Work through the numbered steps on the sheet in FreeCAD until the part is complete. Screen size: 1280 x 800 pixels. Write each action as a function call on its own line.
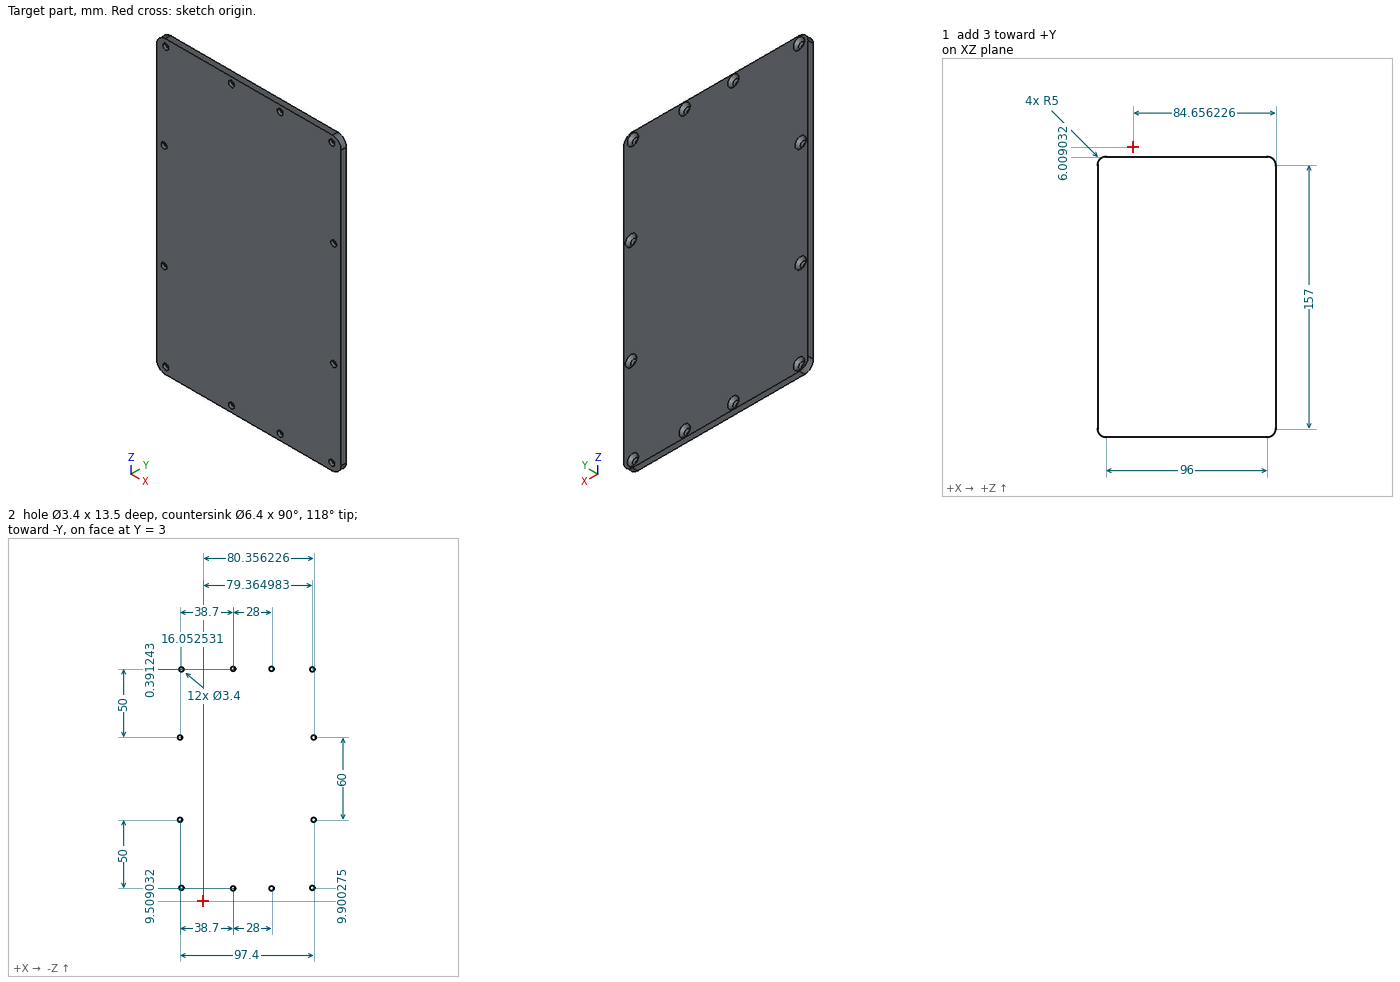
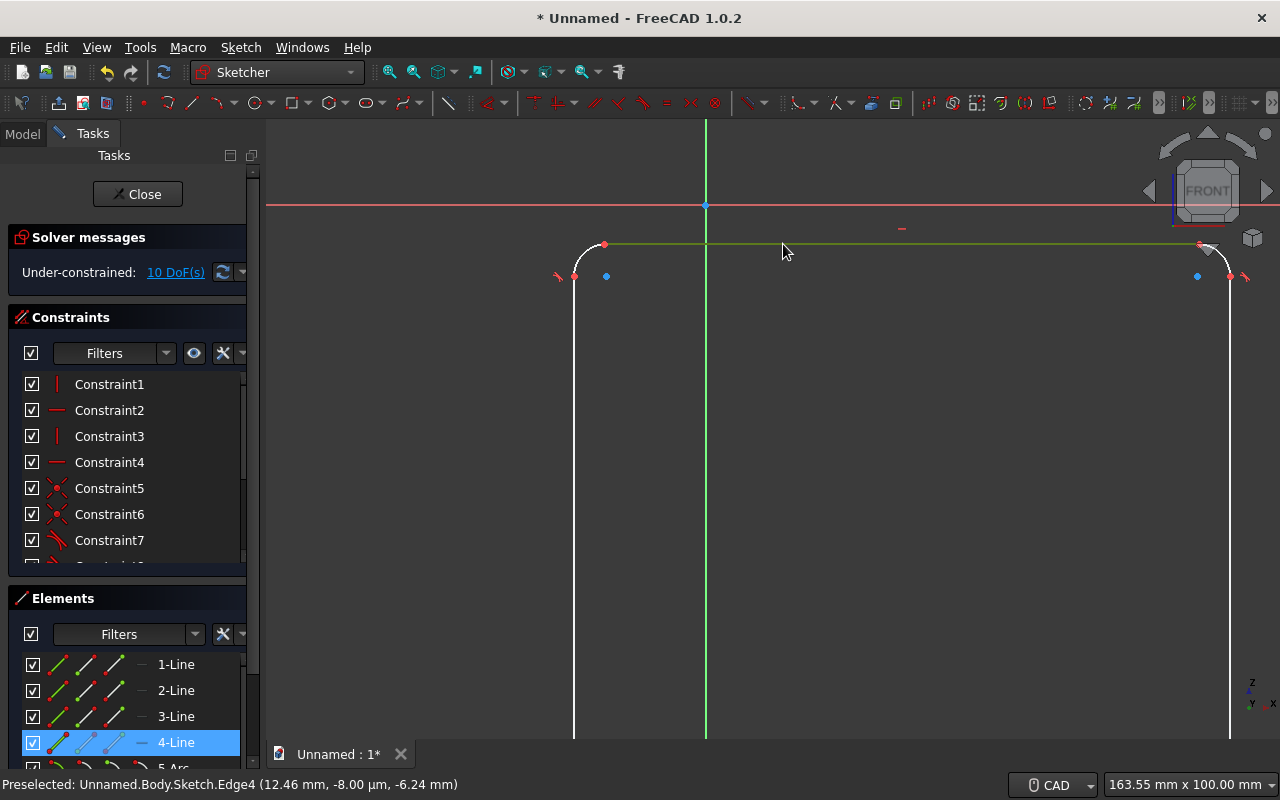
click(591, 248)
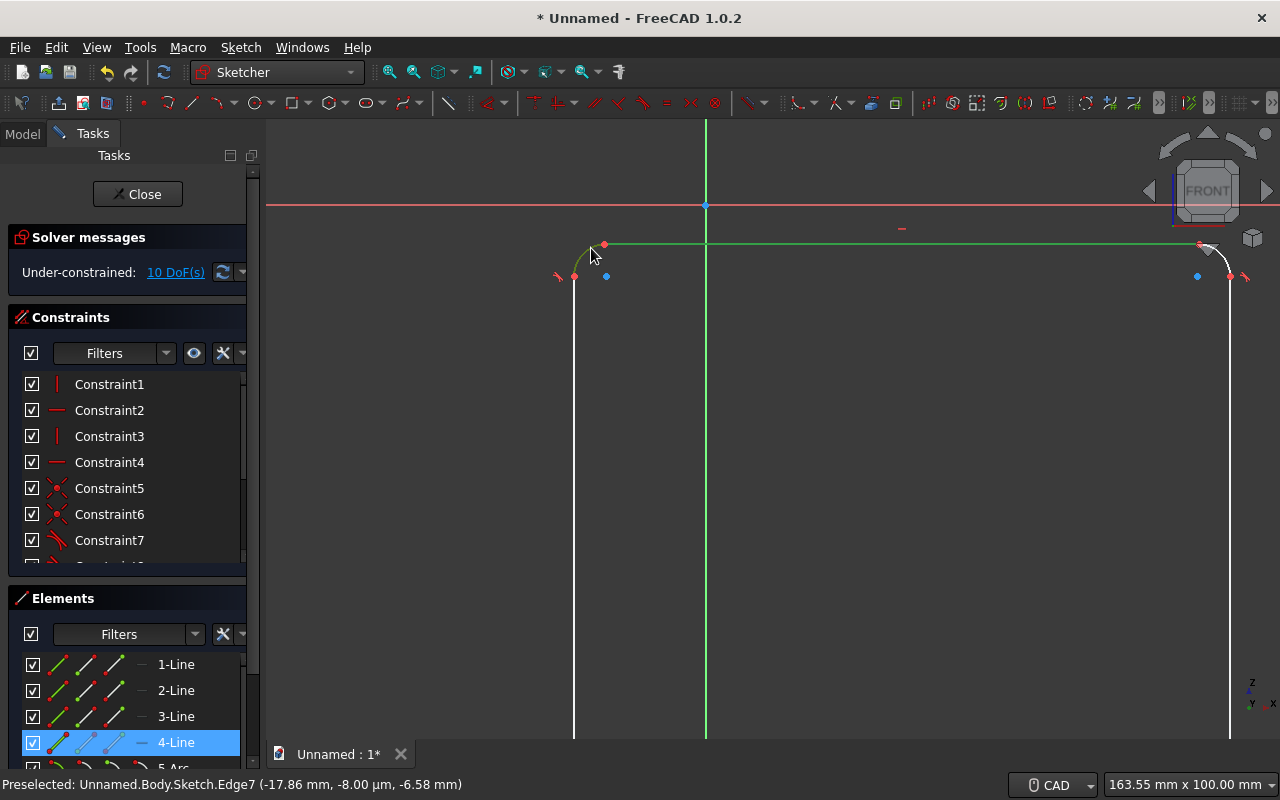
click(644, 104)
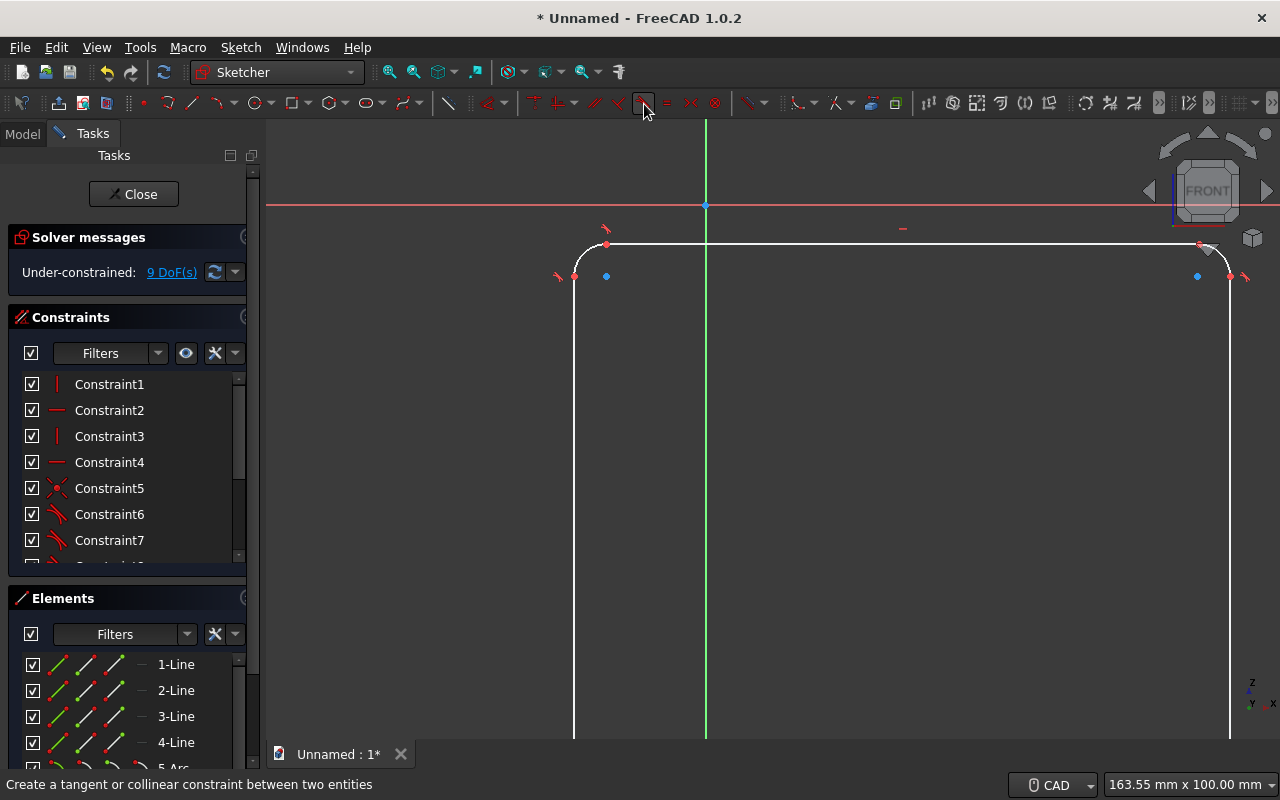
click(785, 244)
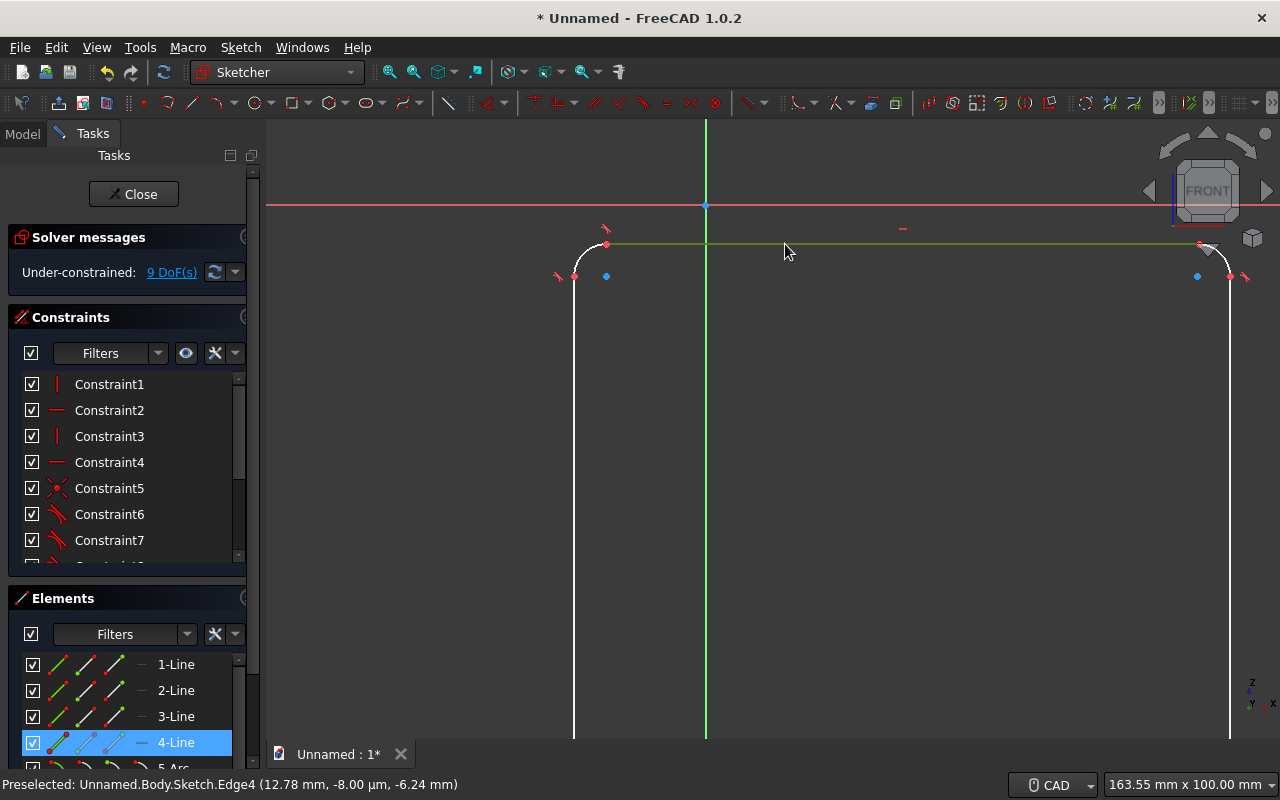
scroll(590, 247, down, 5)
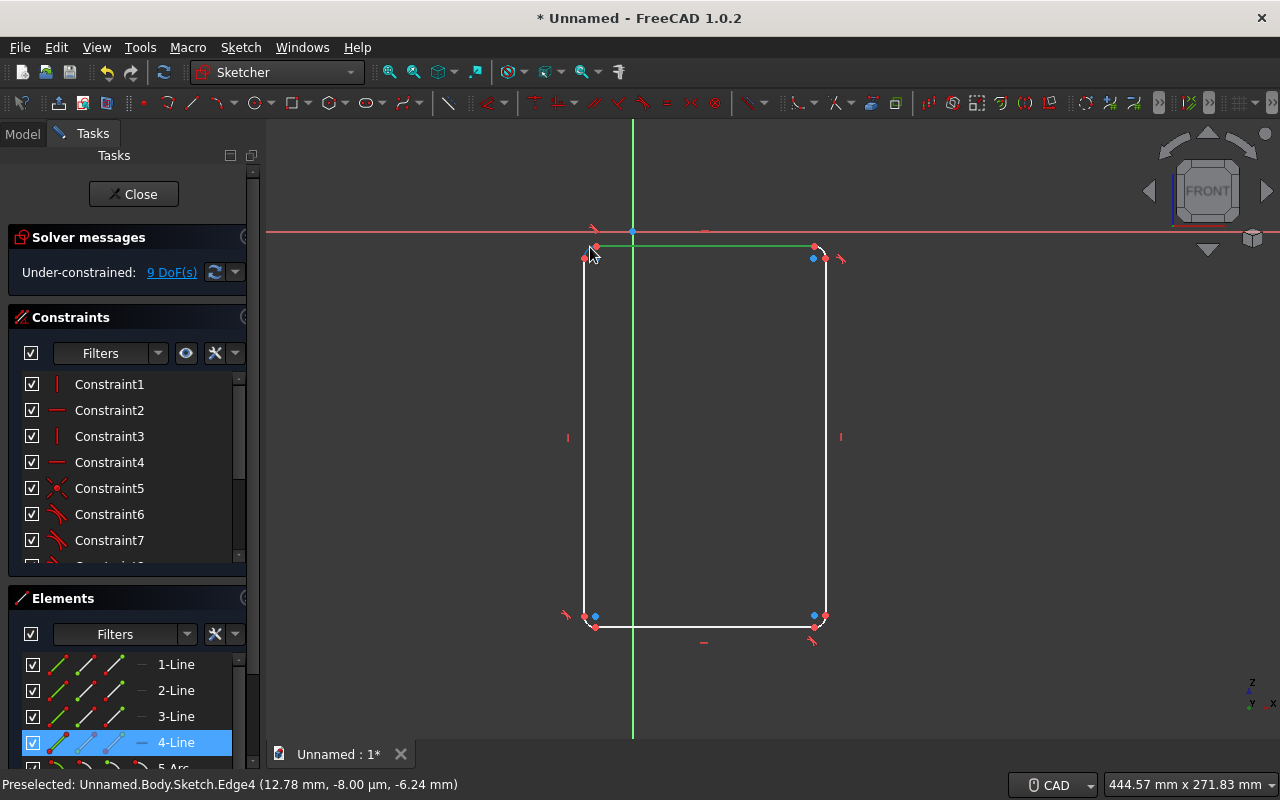
scroll(825, 253, up, 5)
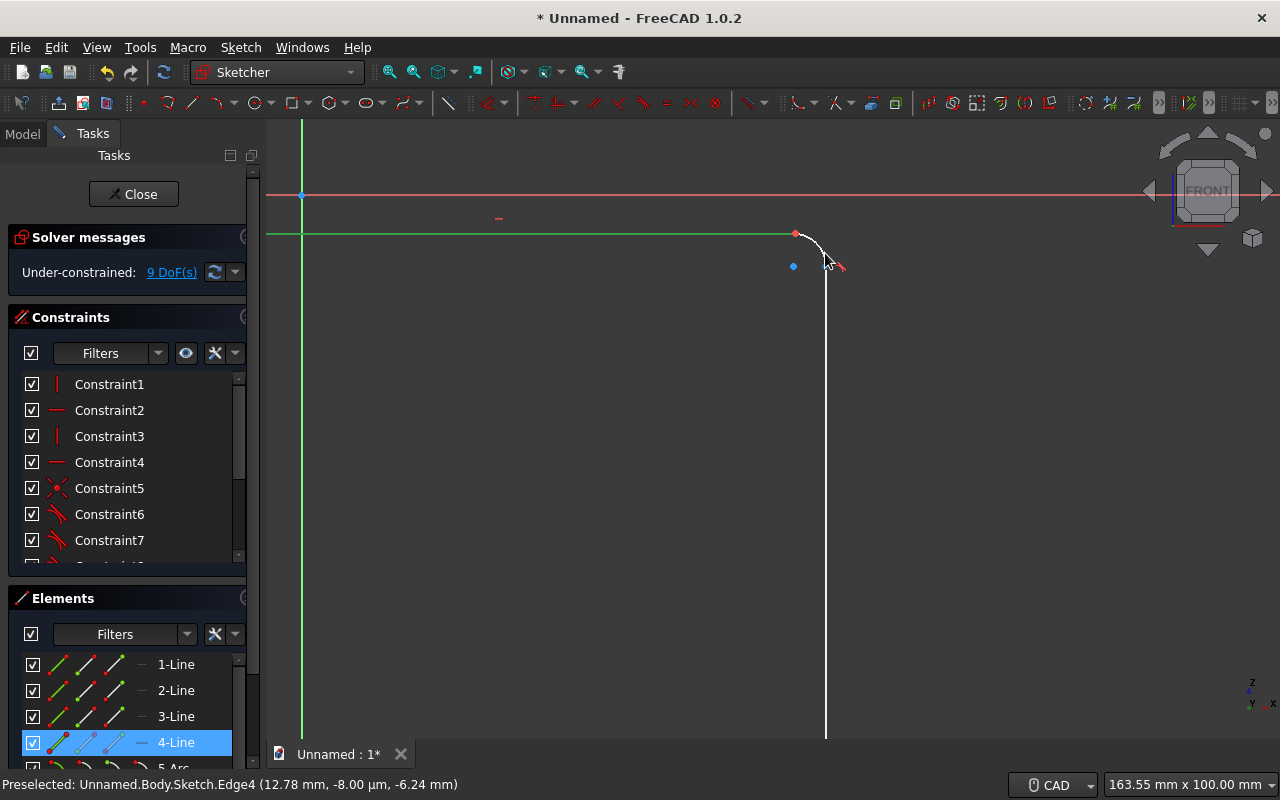
click(823, 252)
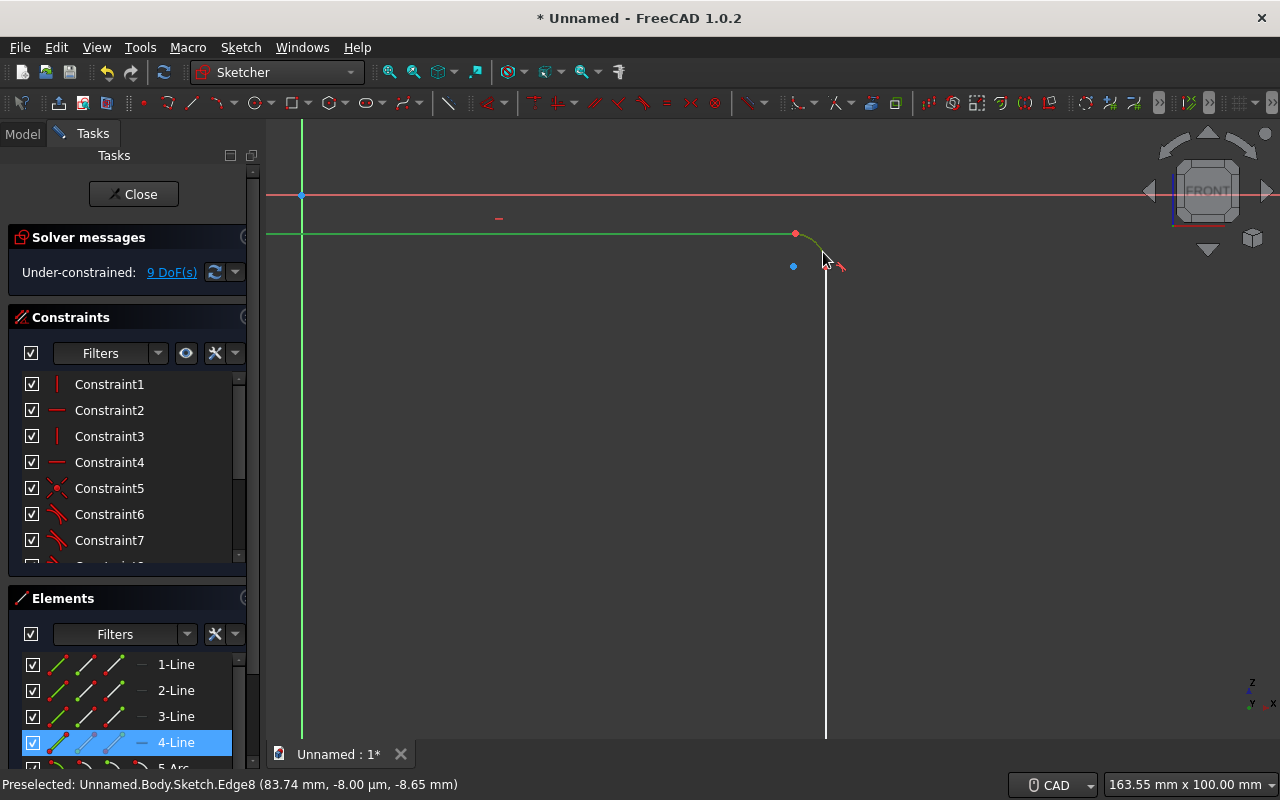
click(644, 104)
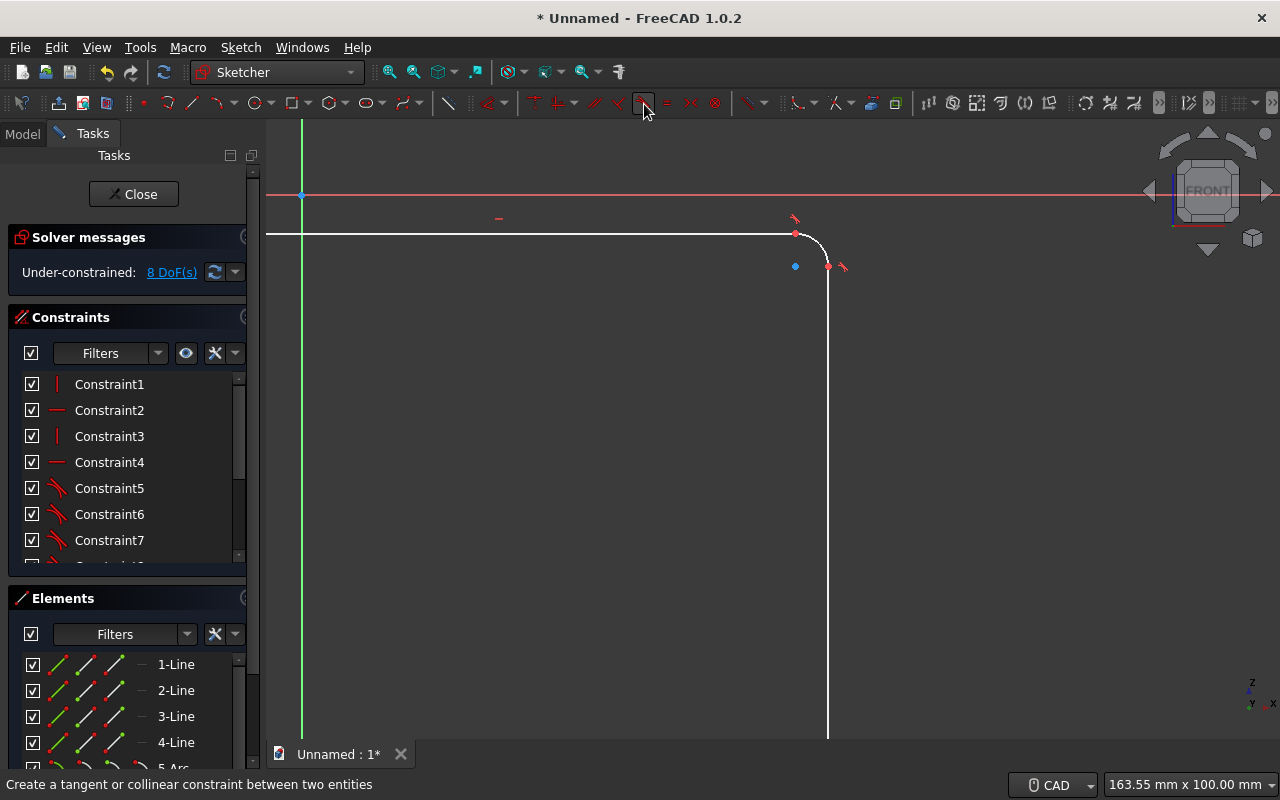
scroll(825, 253, down, 5)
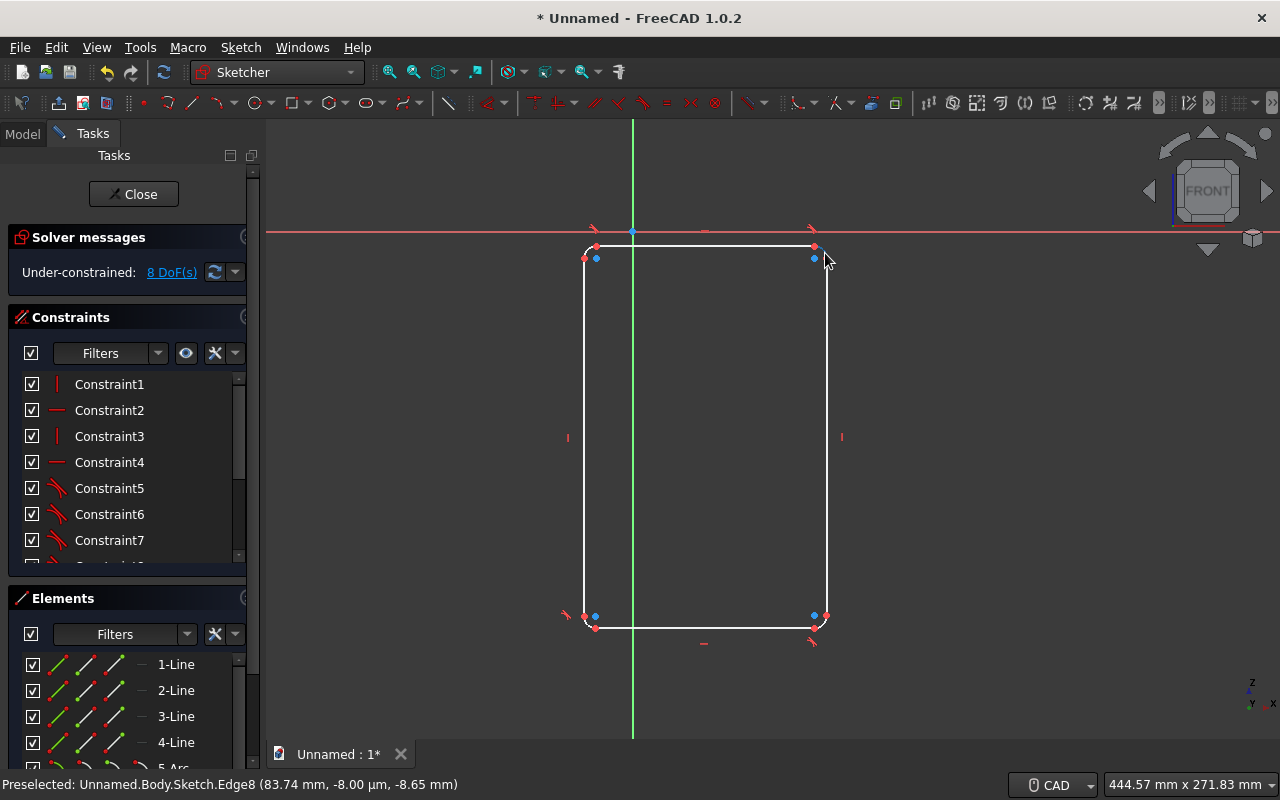
scroll(820, 627, up, 5)